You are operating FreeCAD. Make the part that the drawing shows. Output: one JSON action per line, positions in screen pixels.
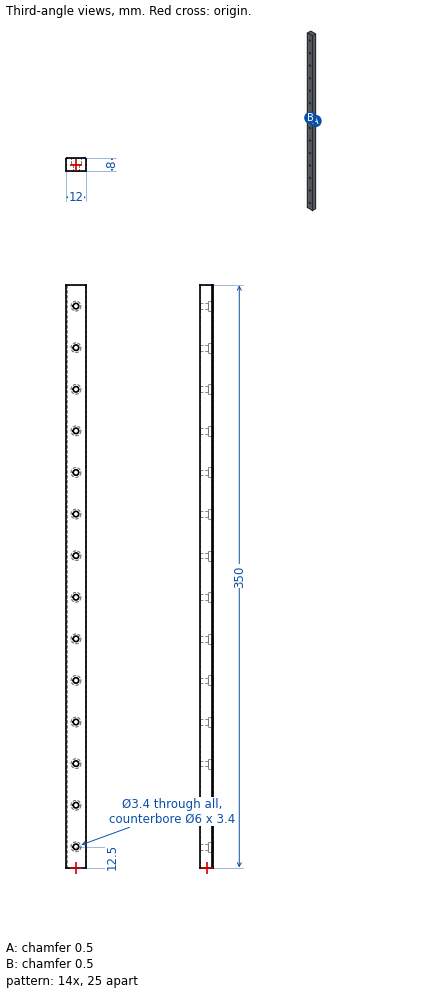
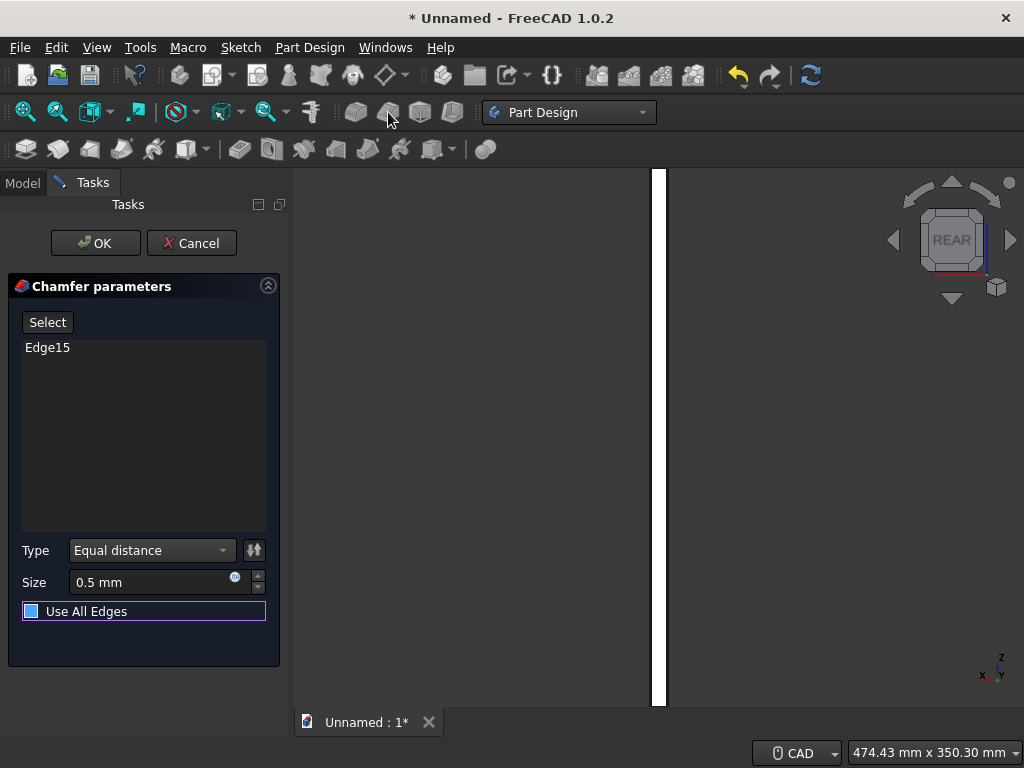
{"action": "left_click", "coordinate": [96, 243]}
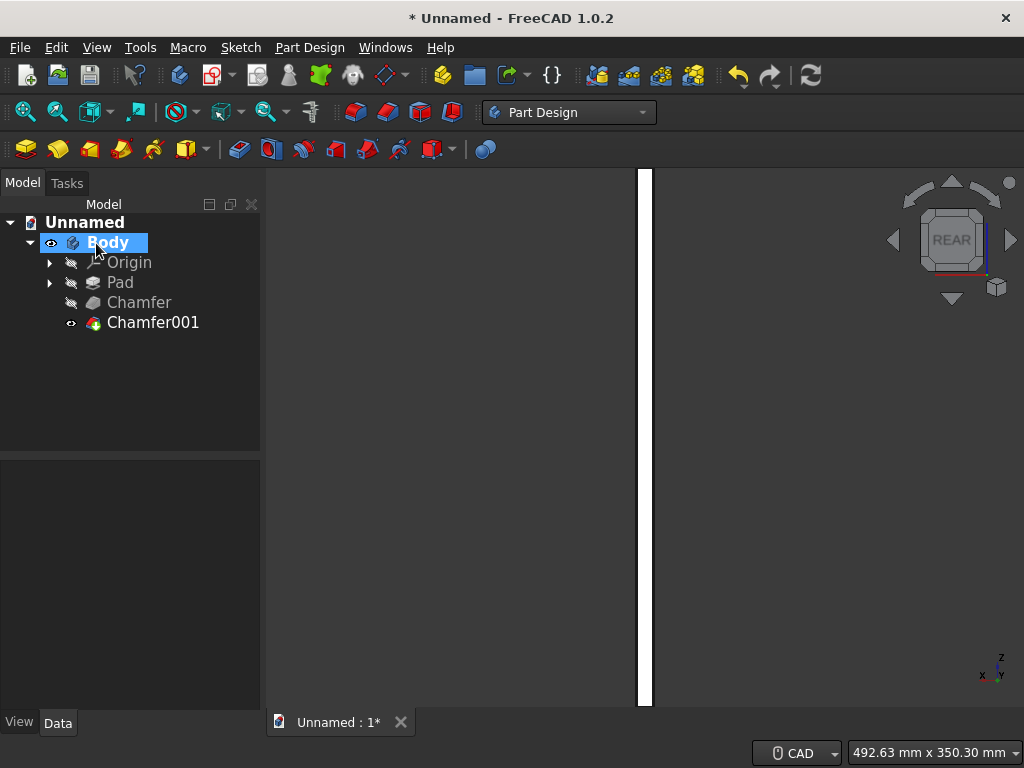
{"action": "left_click", "coordinate": [26, 112]}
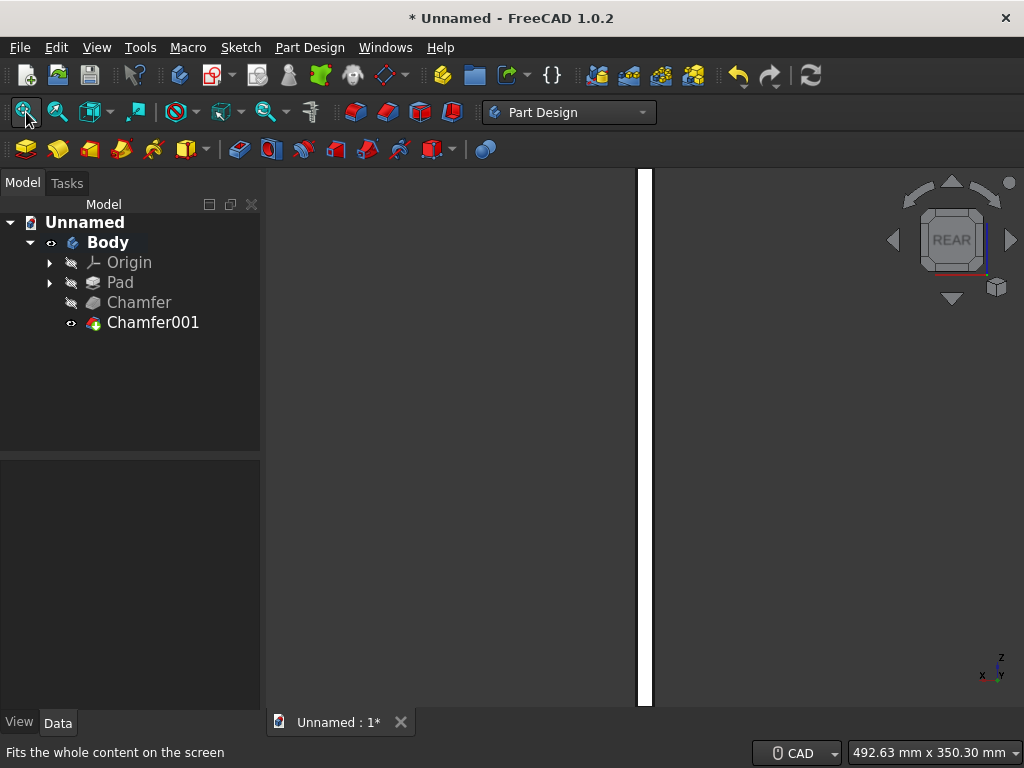
{"action": "left_click", "coordinate": [645, 206]}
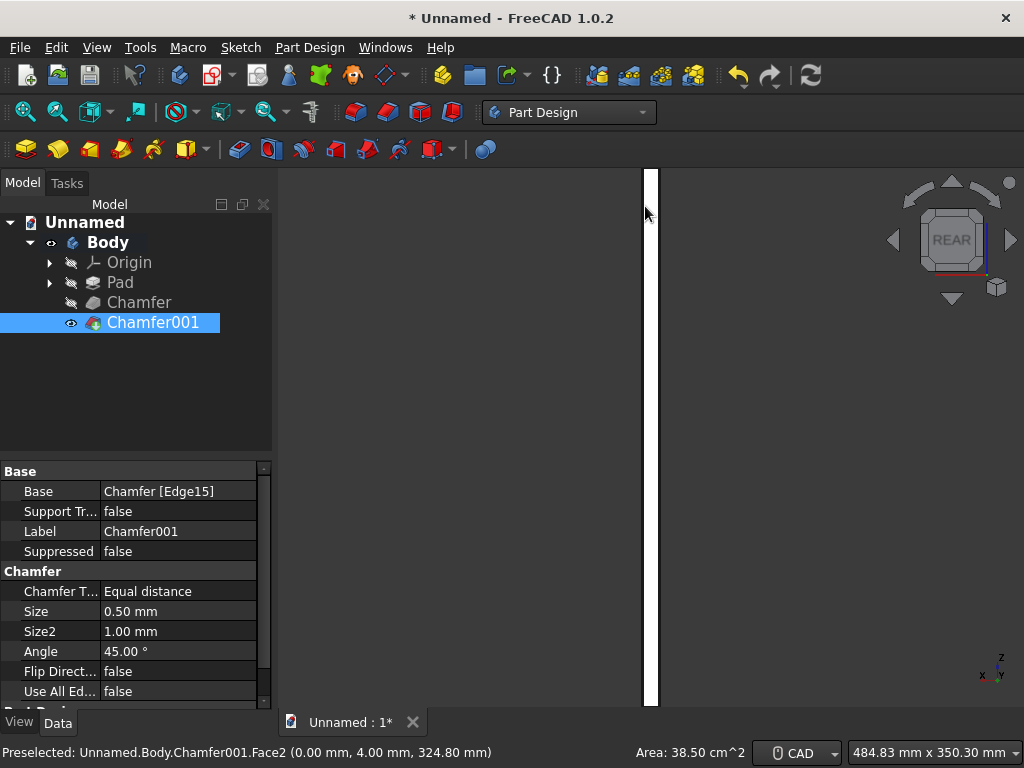
{"action": "left_click", "coordinate": [212, 76]}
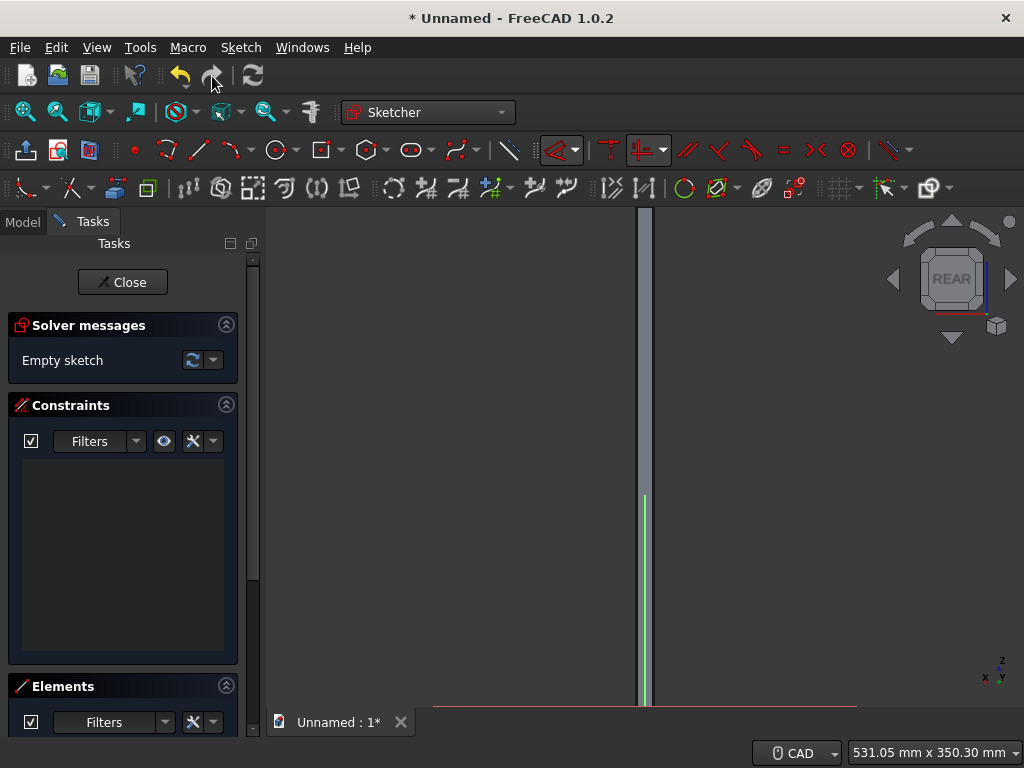
{"action": "scroll", "coordinate": [576, 457], "scroll_direction": "down", "scroll_amount": 5}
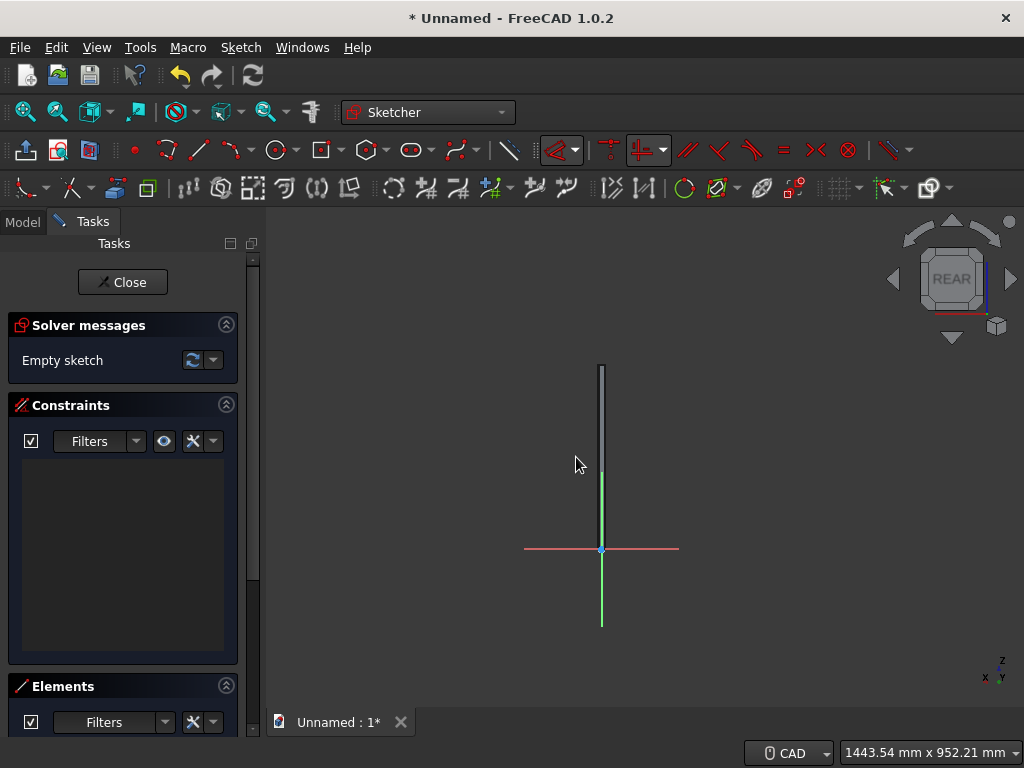
{"action": "scroll", "coordinate": [603, 547], "scroll_direction": "up", "scroll_amount": 15}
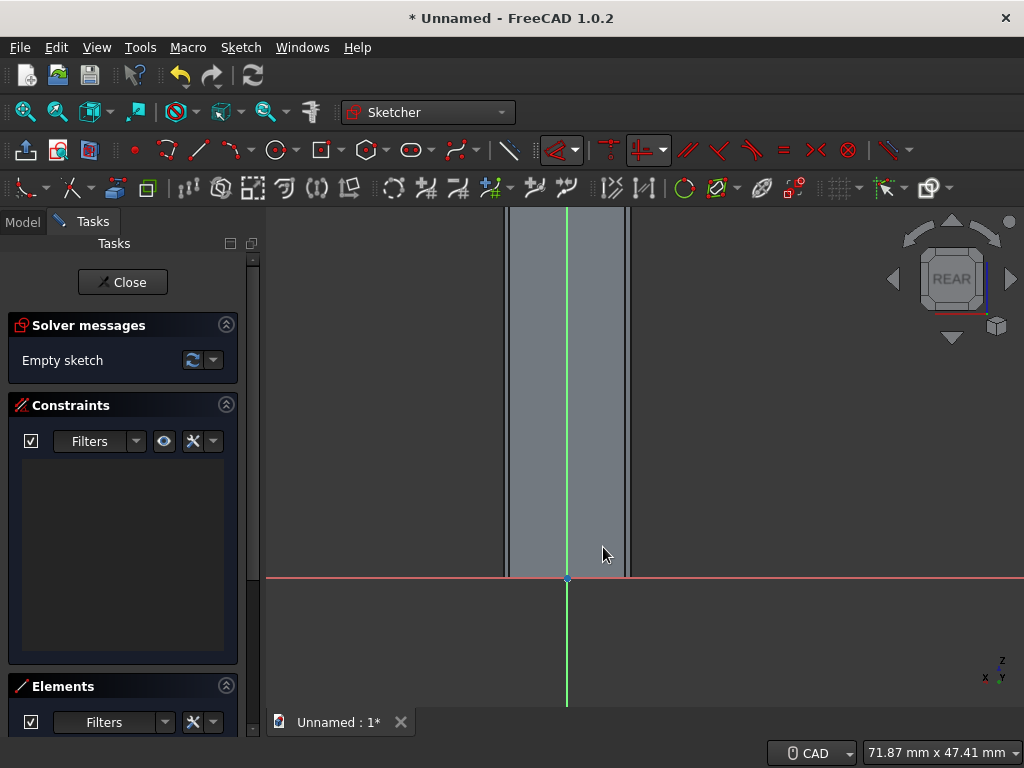
{"action": "scroll", "coordinate": [566, 445], "scroll_direction": "up", "scroll_amount": 11}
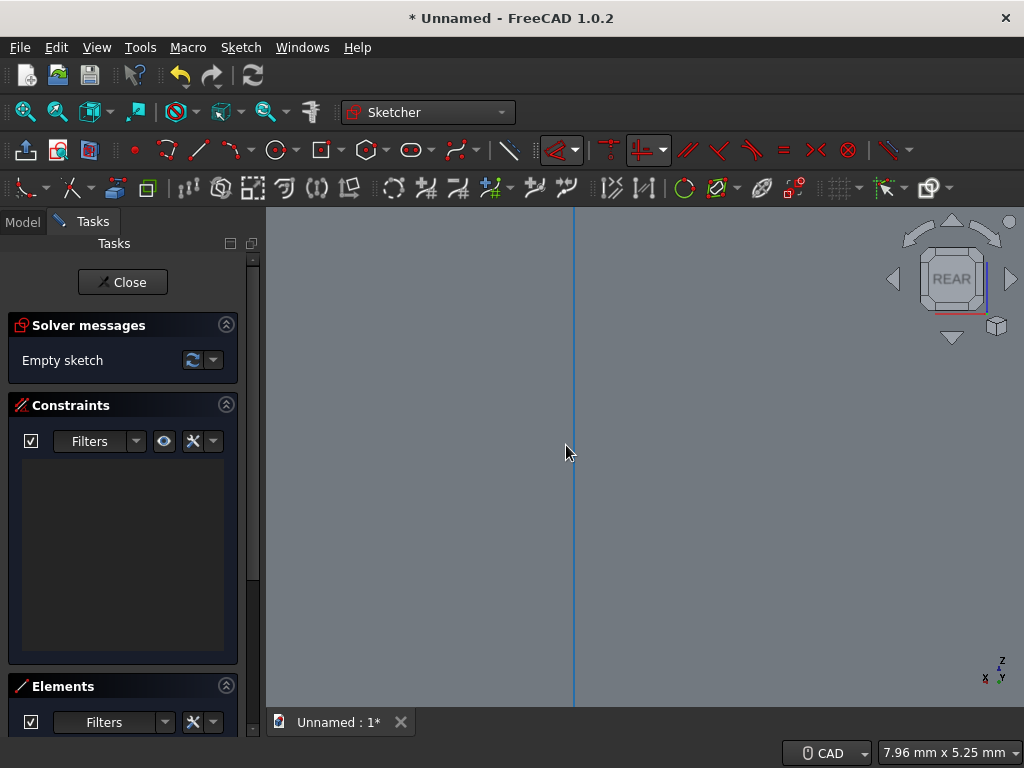
{"action": "left_click", "coordinate": [276, 150]}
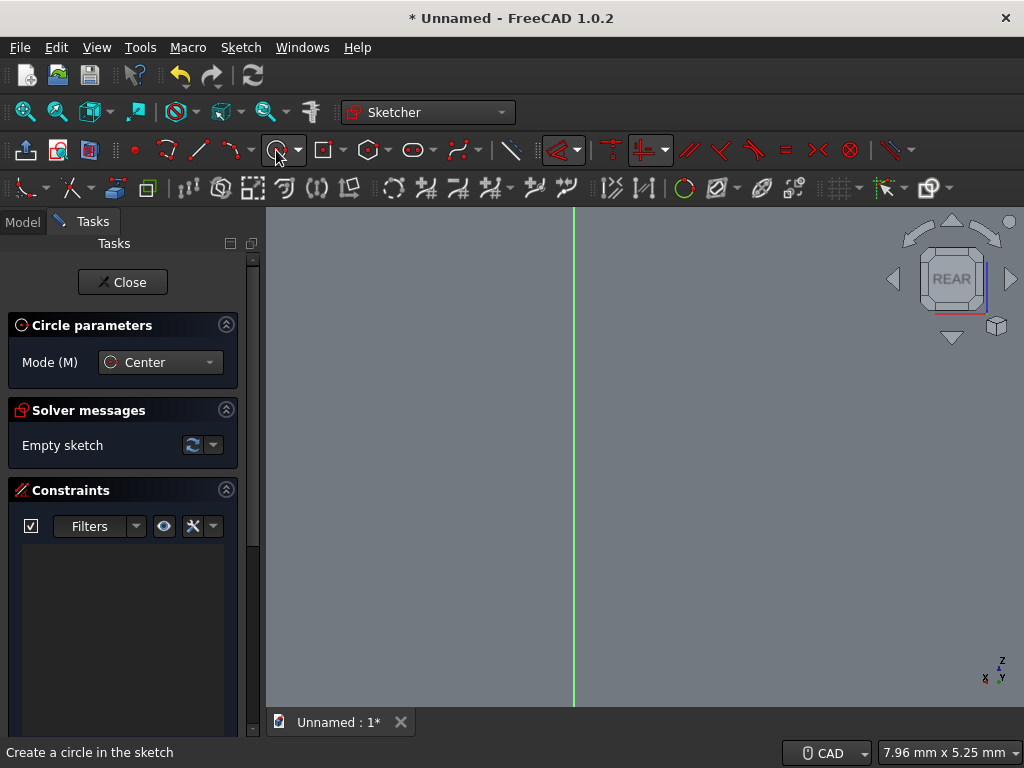
{"action": "left_click", "coordinate": [574, 455]}
{"action": "mouse_move", "coordinate": [688, 340]}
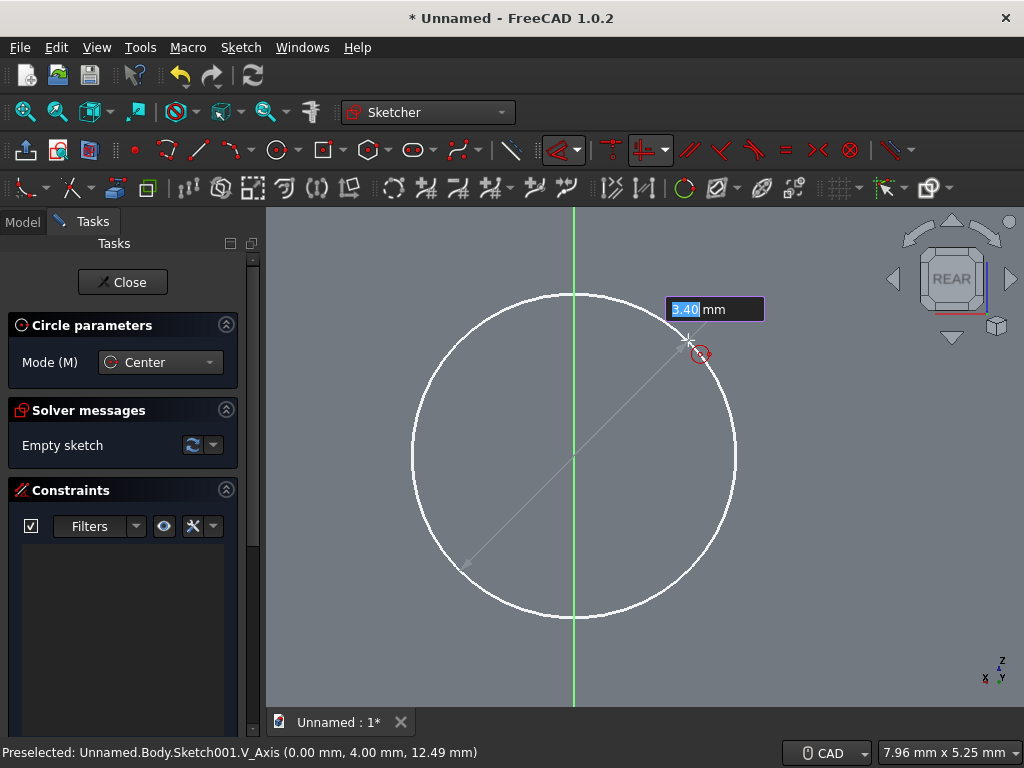
{"action": "type", "text": "3.4"}
{"action": "key", "text": "Return"}
{"action": "key", "text": "Escape"}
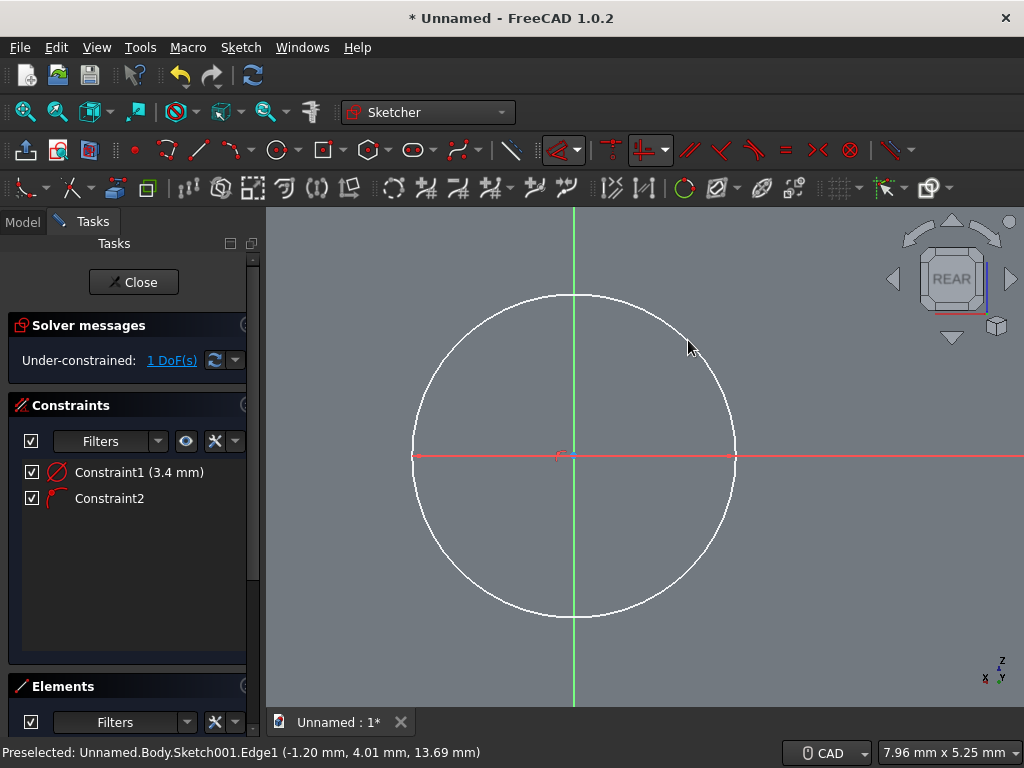
{"action": "left_click", "coordinate": [558, 150]}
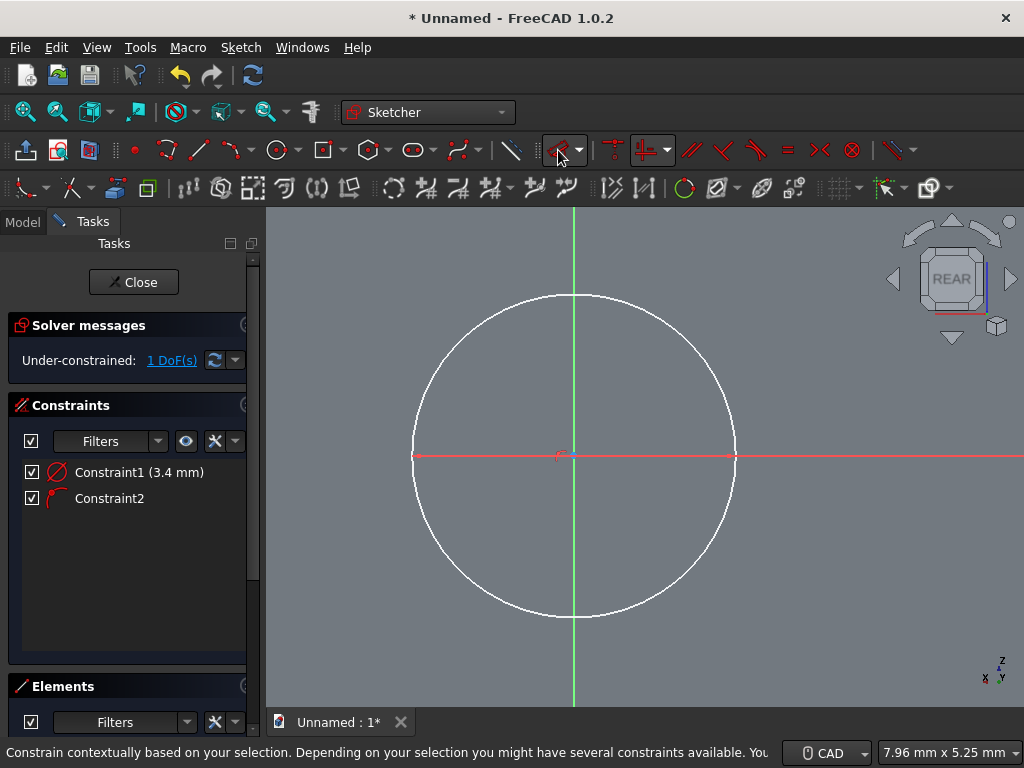
{"action": "left_click", "coordinate": [574, 456]}
{"action": "left_click", "coordinate": [608, 568]}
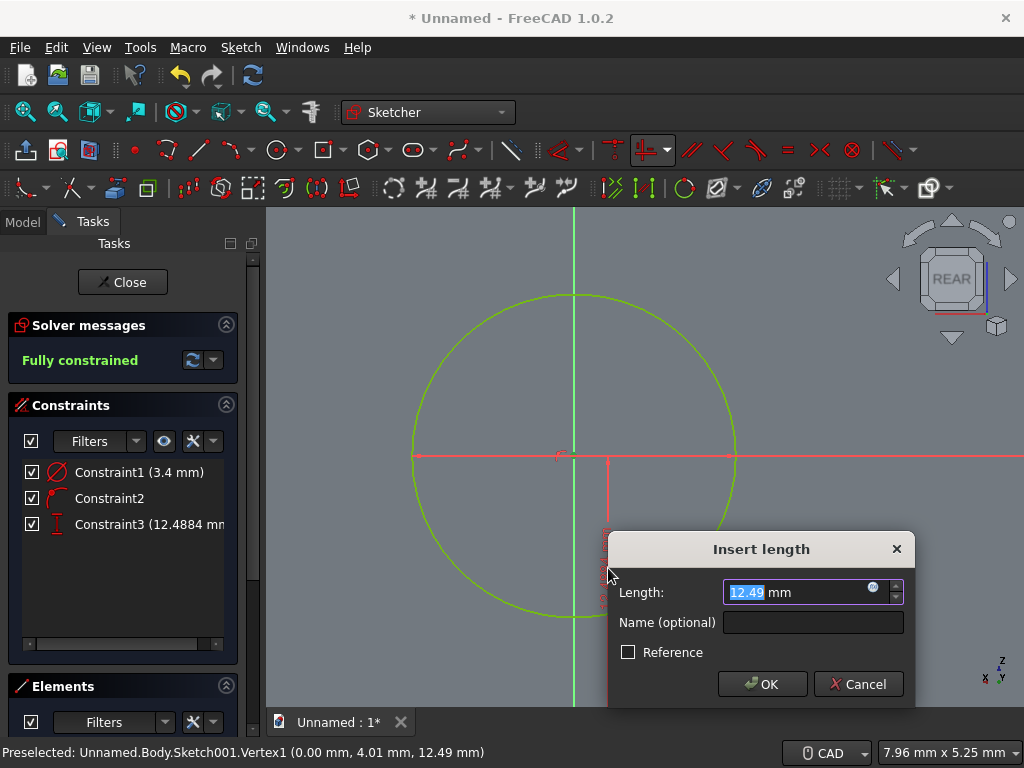
{"action": "type", "text": "12.5"}
{"action": "key", "text": "Return"}
{"action": "key", "text": "Escape"}